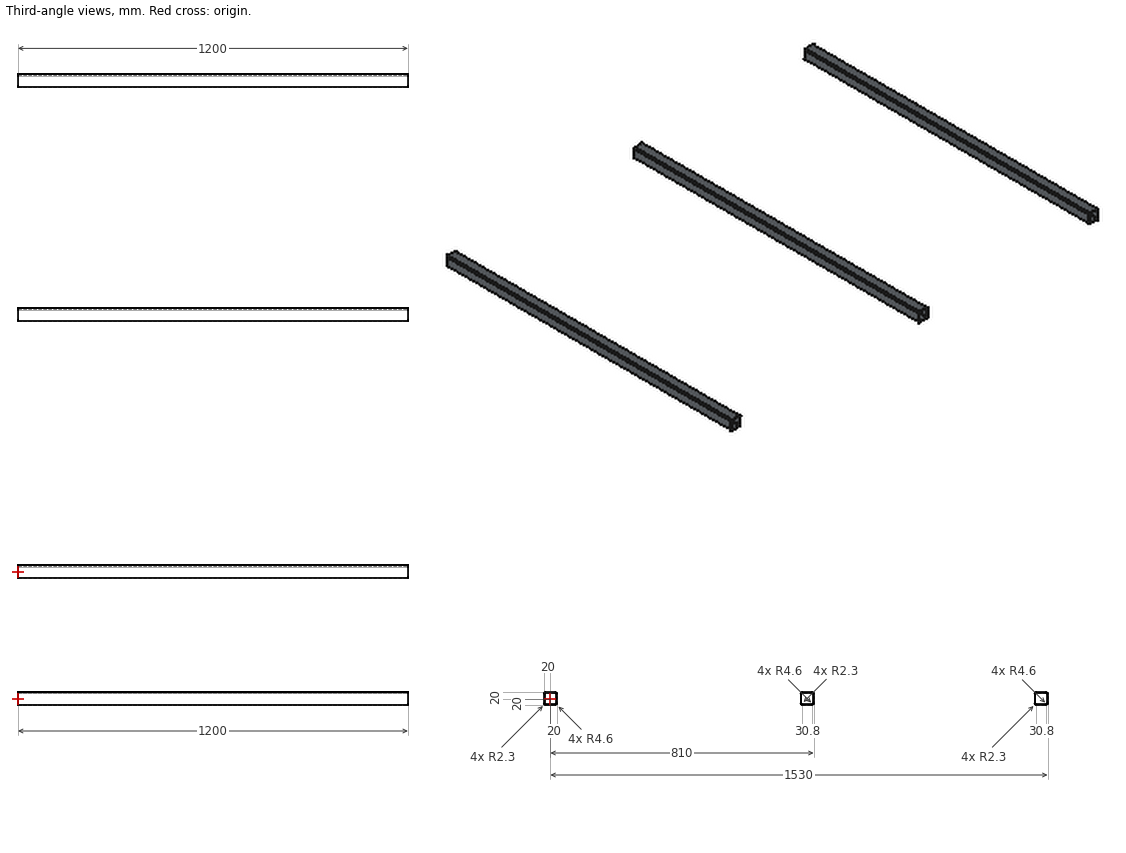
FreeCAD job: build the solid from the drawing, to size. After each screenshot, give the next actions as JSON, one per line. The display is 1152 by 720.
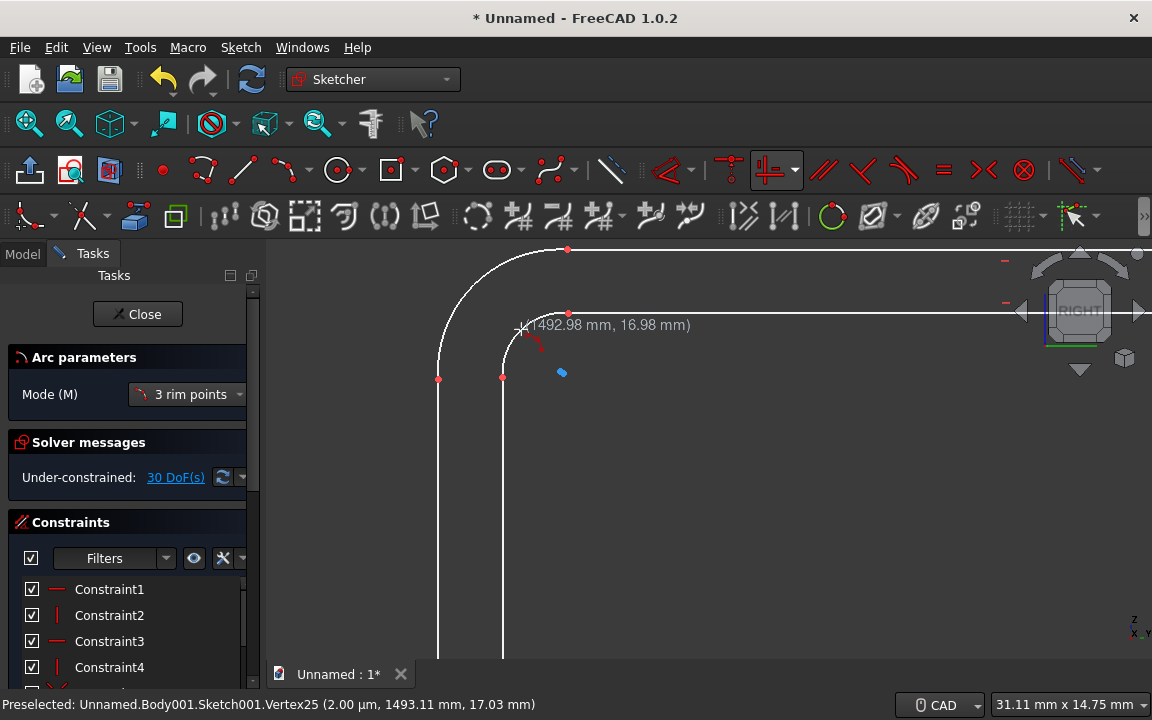
{"action": "scroll", "coordinate": [521, 330], "scroll_direction": "down", "scroll_amount": 7}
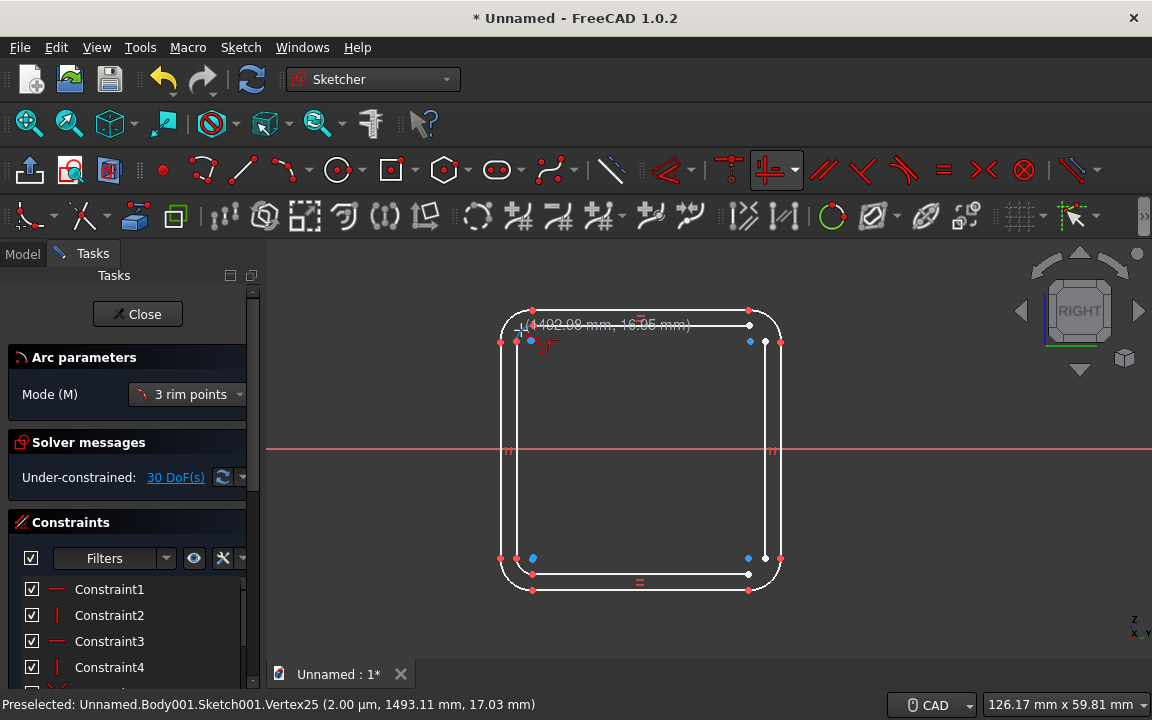
{"action": "left_click", "coordinate": [749, 326]}
{"action": "left_click", "coordinate": [765, 342]}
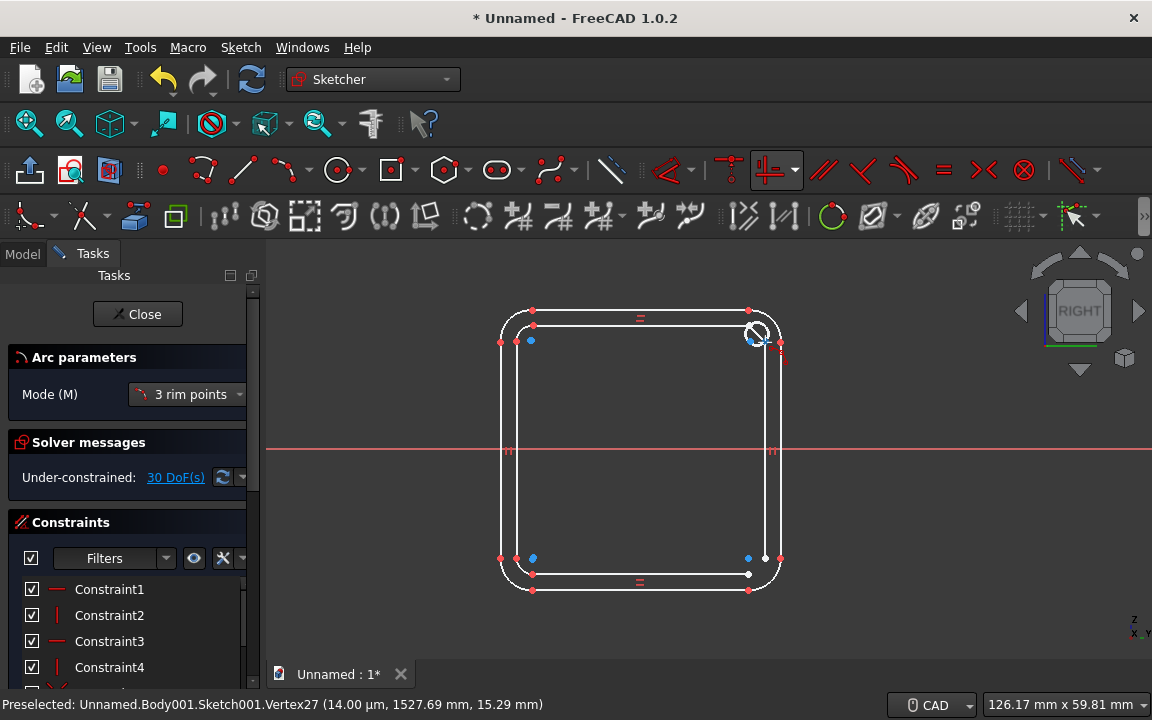
{"action": "scroll", "coordinate": [760, 330], "scroll_direction": "up", "scroll_amount": 7}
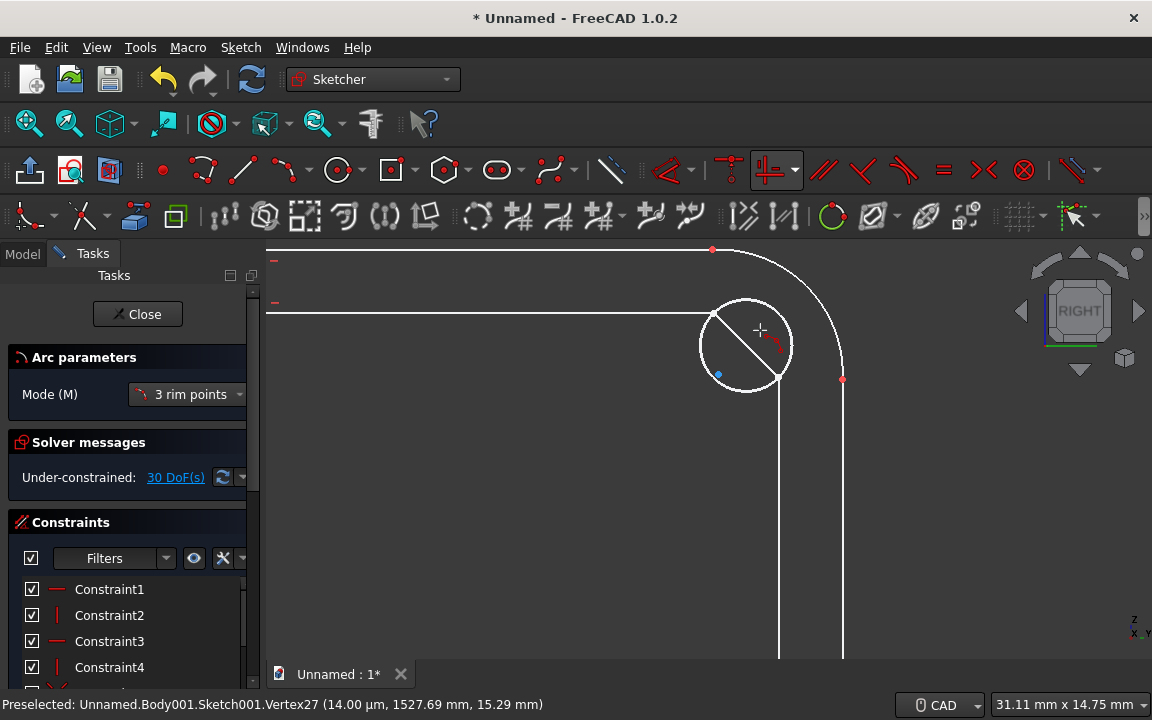
{"action": "left_click", "coordinate": [760, 329]}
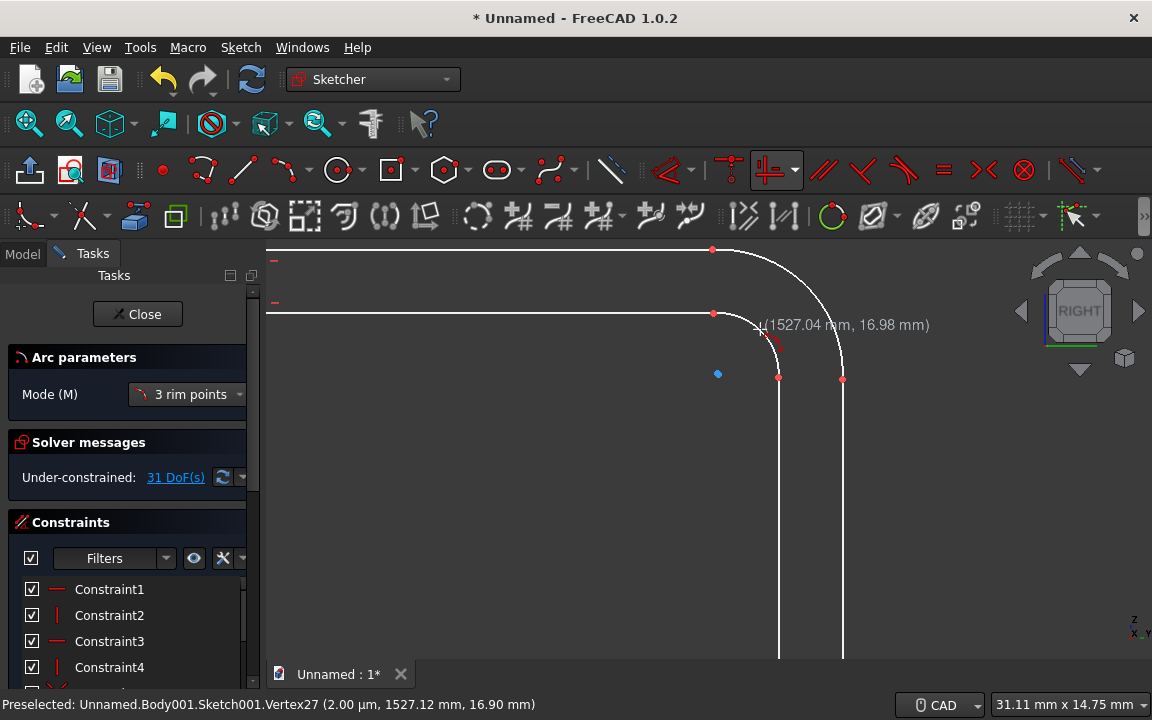
{"action": "scroll", "coordinate": [760, 330], "scroll_direction": "down", "scroll_amount": 7}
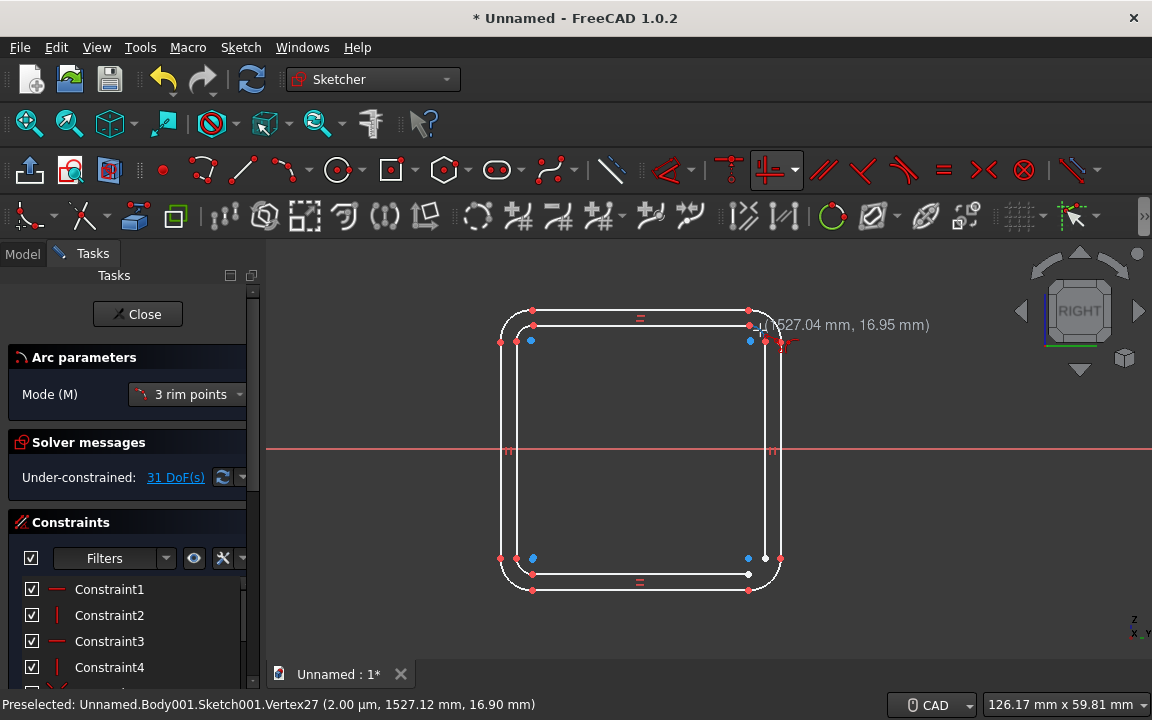
{"action": "left_click", "coordinate": [765, 559]}
{"action": "left_click", "coordinate": [749, 574]}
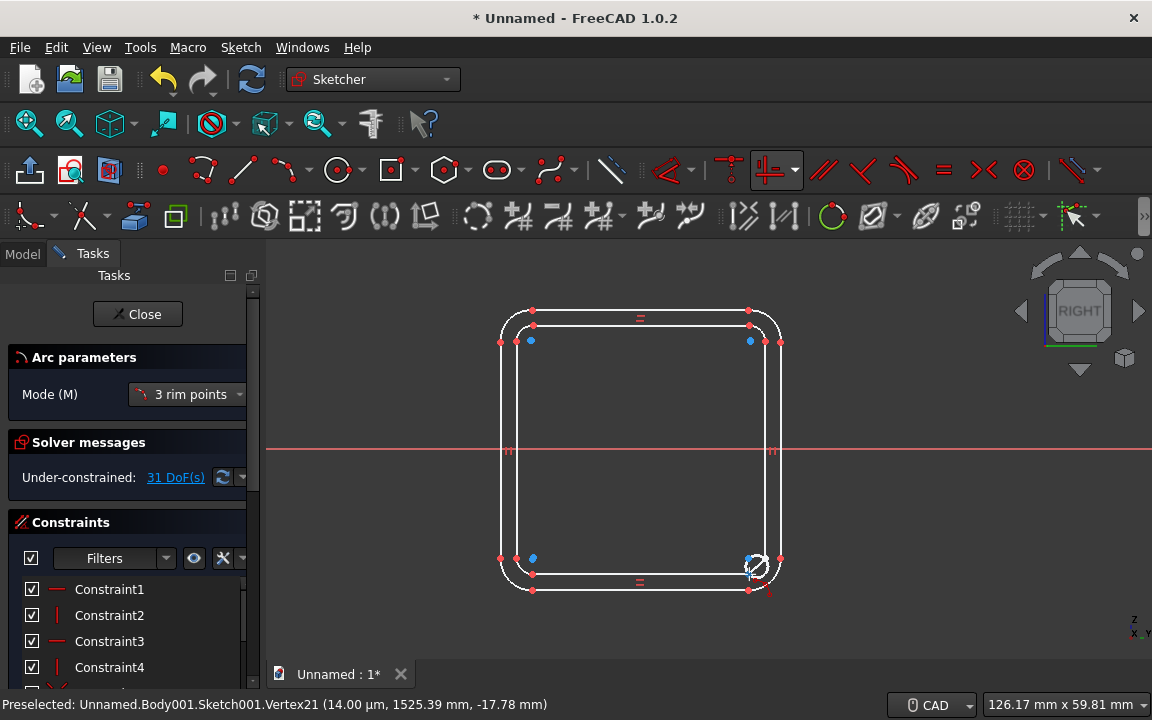
{"action": "scroll", "coordinate": [760, 569], "scroll_direction": "up", "scroll_amount": 7}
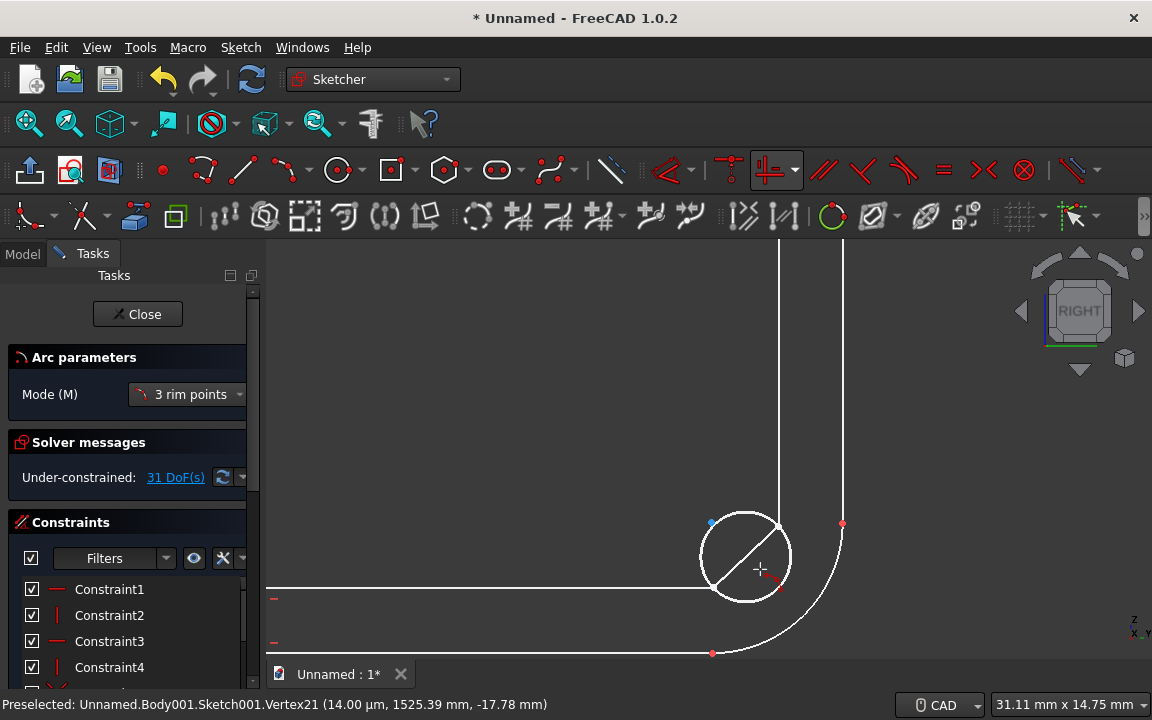
{"action": "left_click", "coordinate": [760, 566]}
{"action": "key", "text": "Escape"}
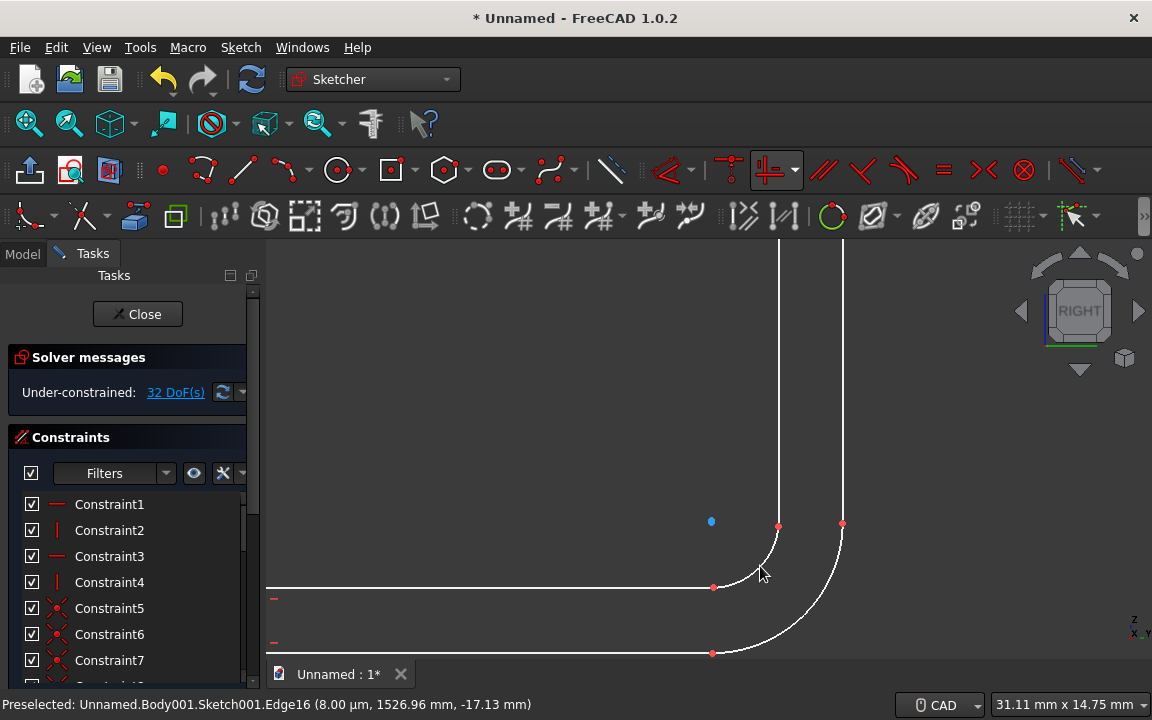
{"action": "scroll", "coordinate": [760, 569], "scroll_direction": "down", "scroll_amount": 7}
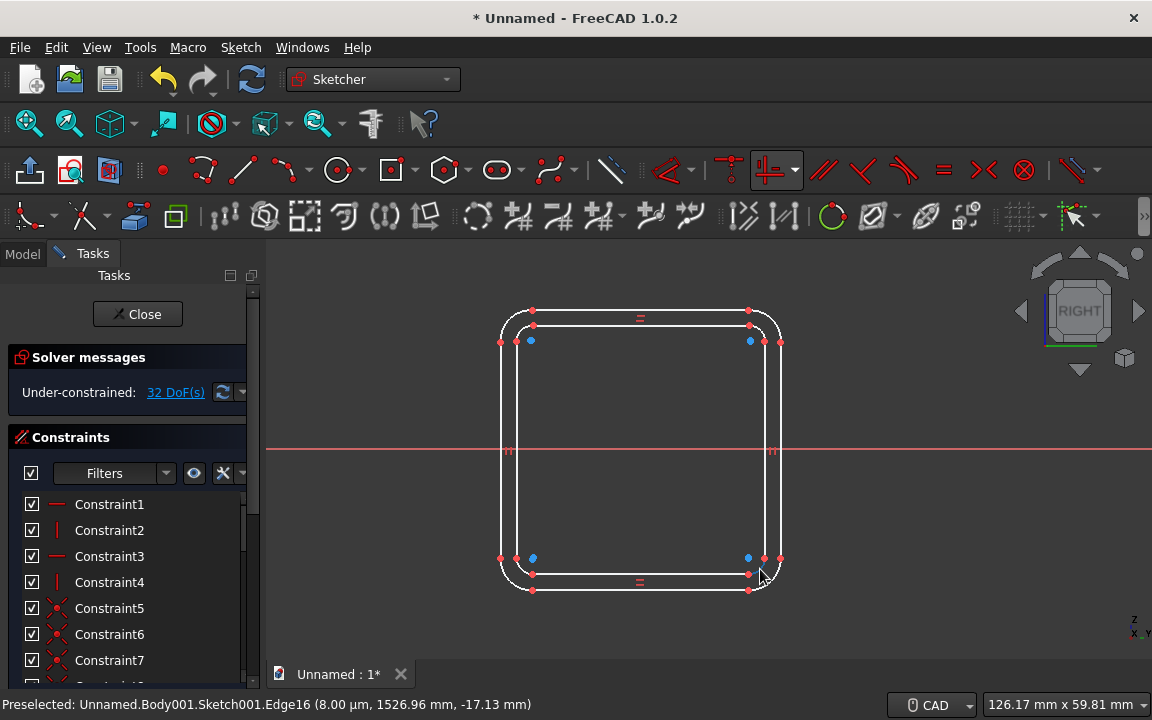
{"action": "left_click", "coordinate": [598, 590]}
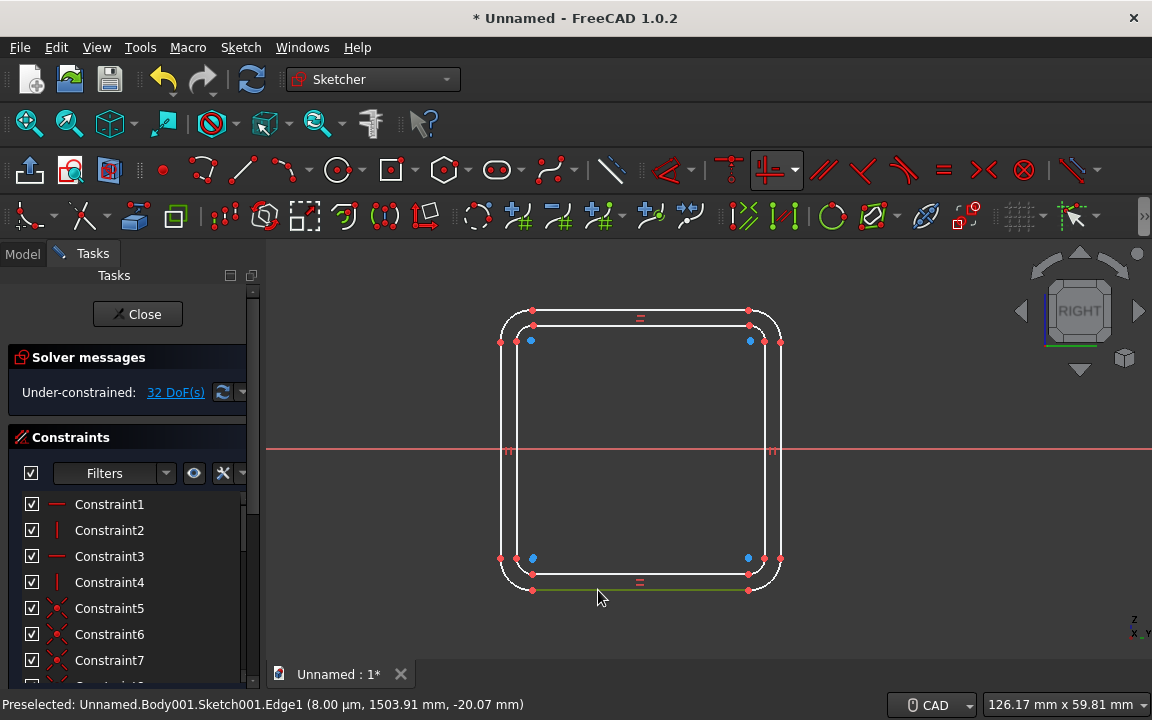
{"action": "left_click", "coordinate": [763, 587]}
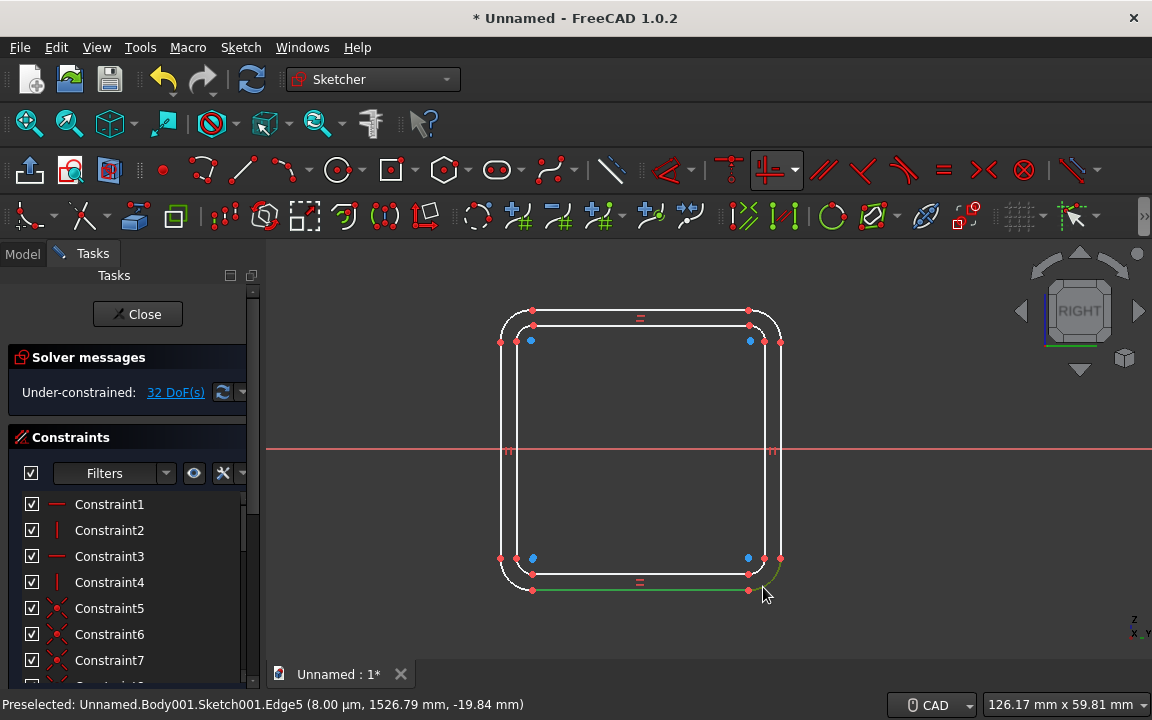
{"action": "key", "text": "t"}